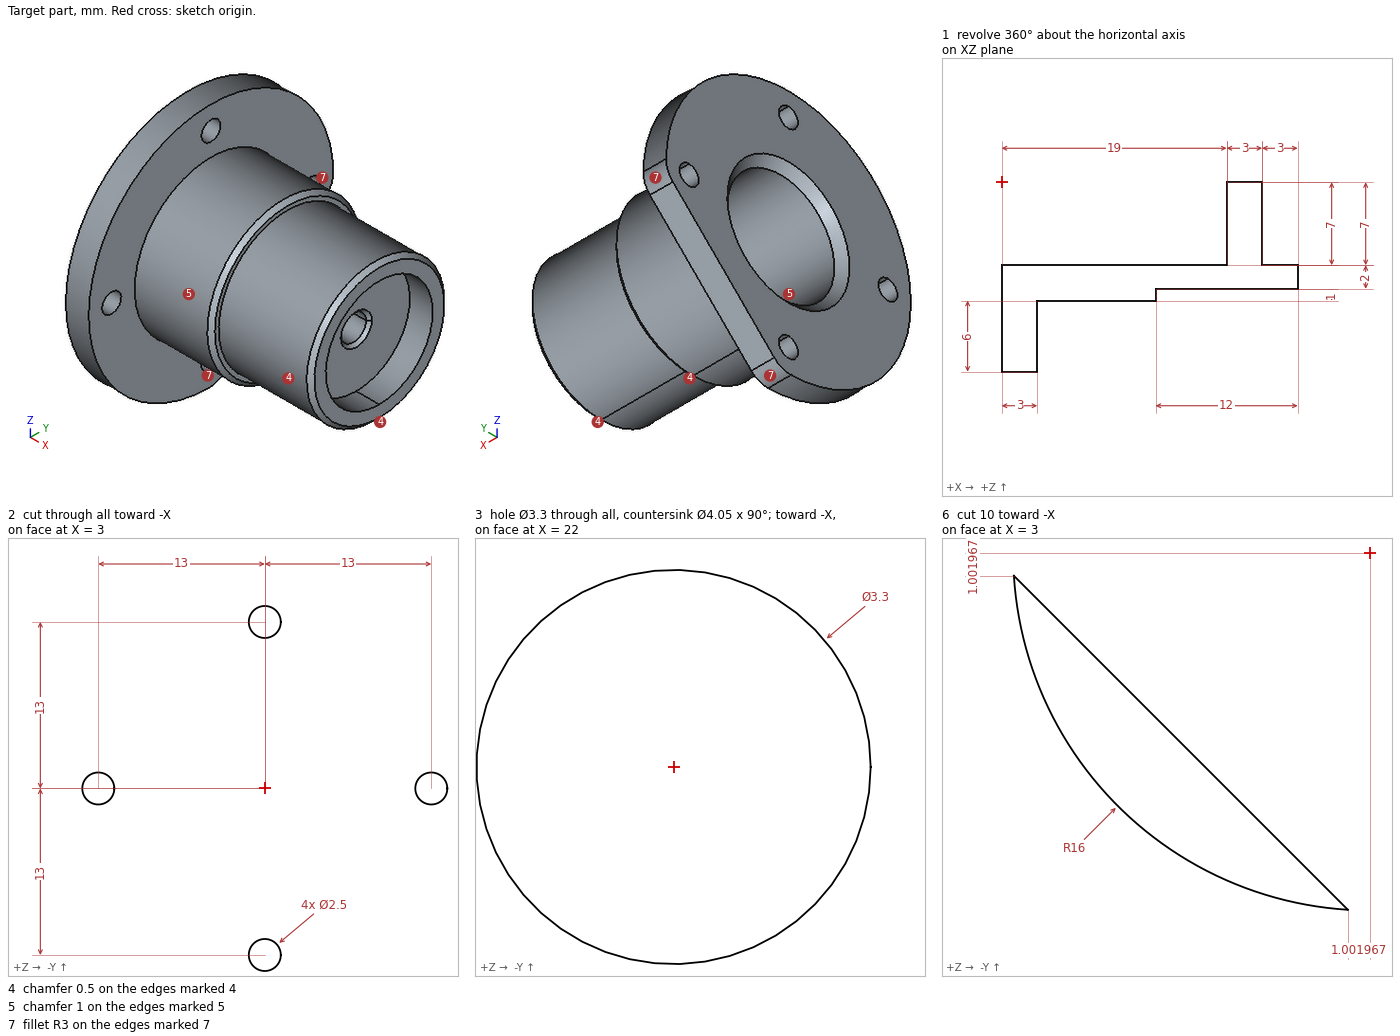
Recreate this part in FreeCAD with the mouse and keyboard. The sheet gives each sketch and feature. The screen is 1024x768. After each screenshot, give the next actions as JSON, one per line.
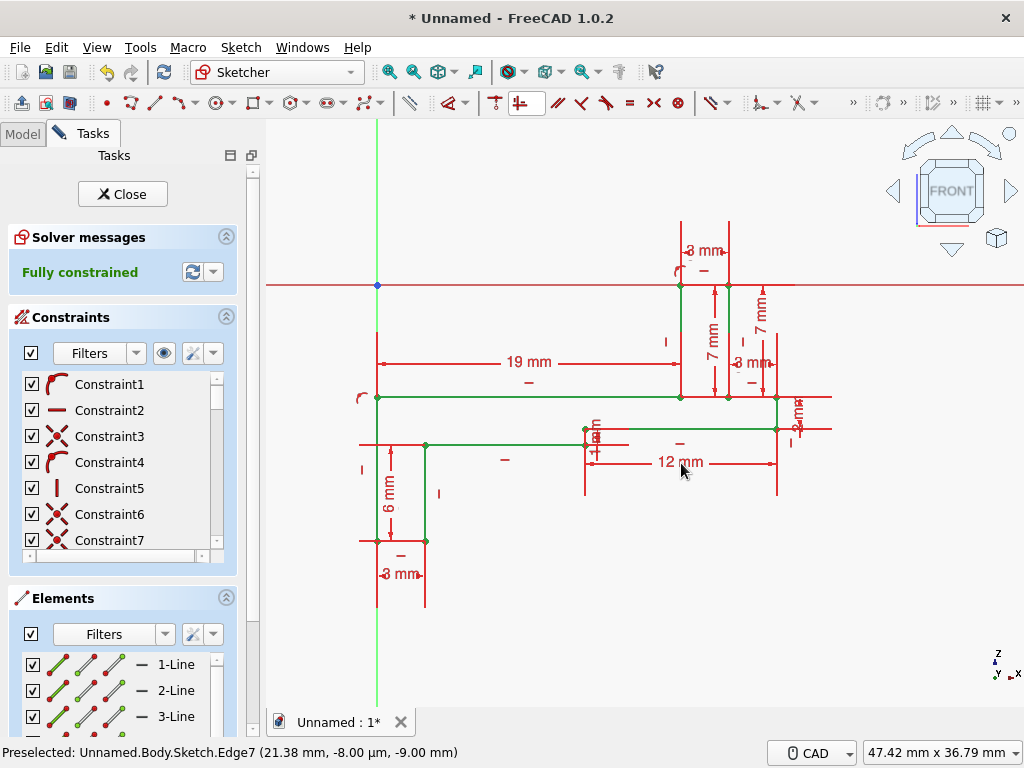
{"action": "left_click", "coordinate": [123, 194]}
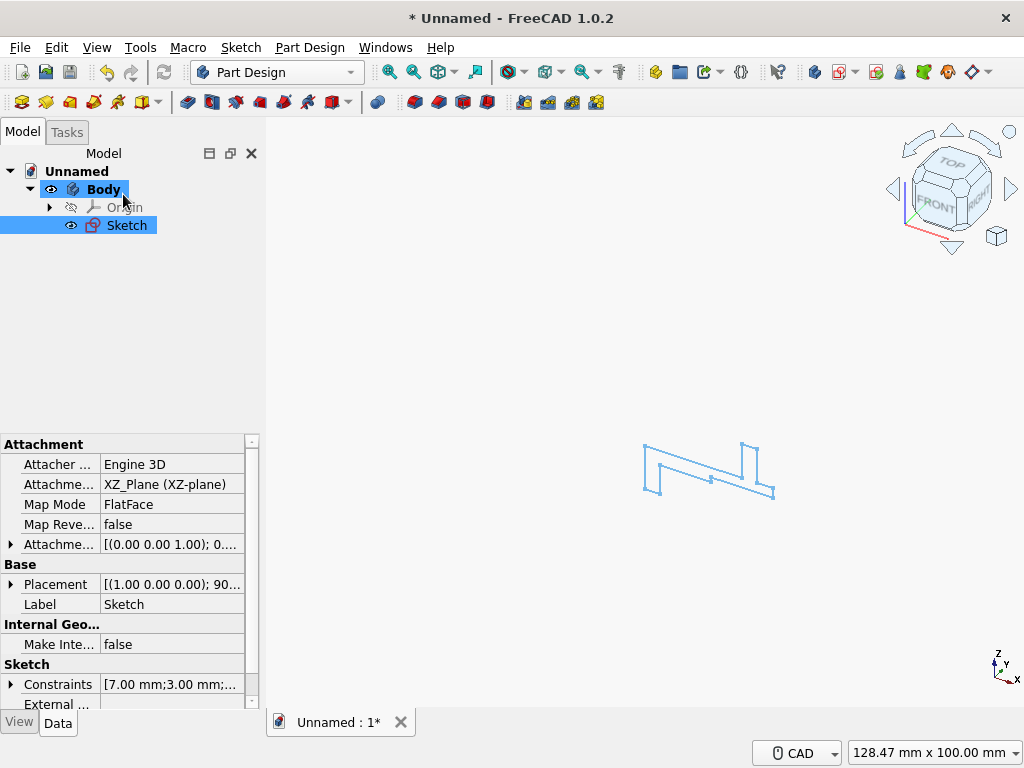
{"action": "left_click", "coordinate": [46, 102]}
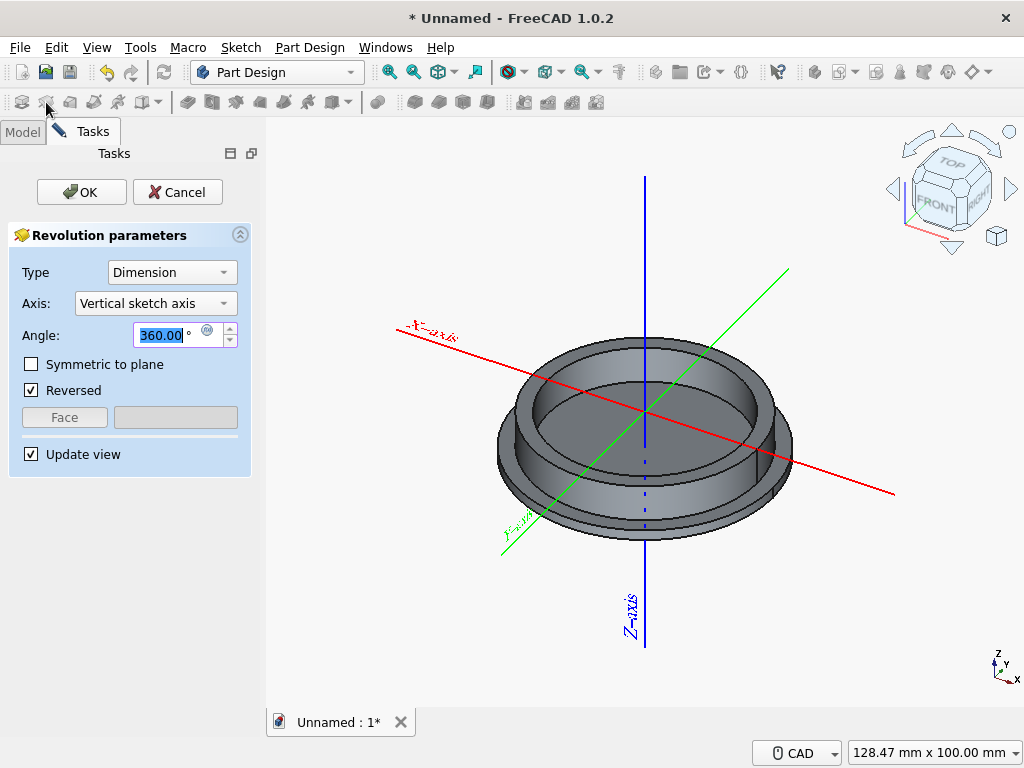
{"action": "left_click", "coordinate": [156, 304]}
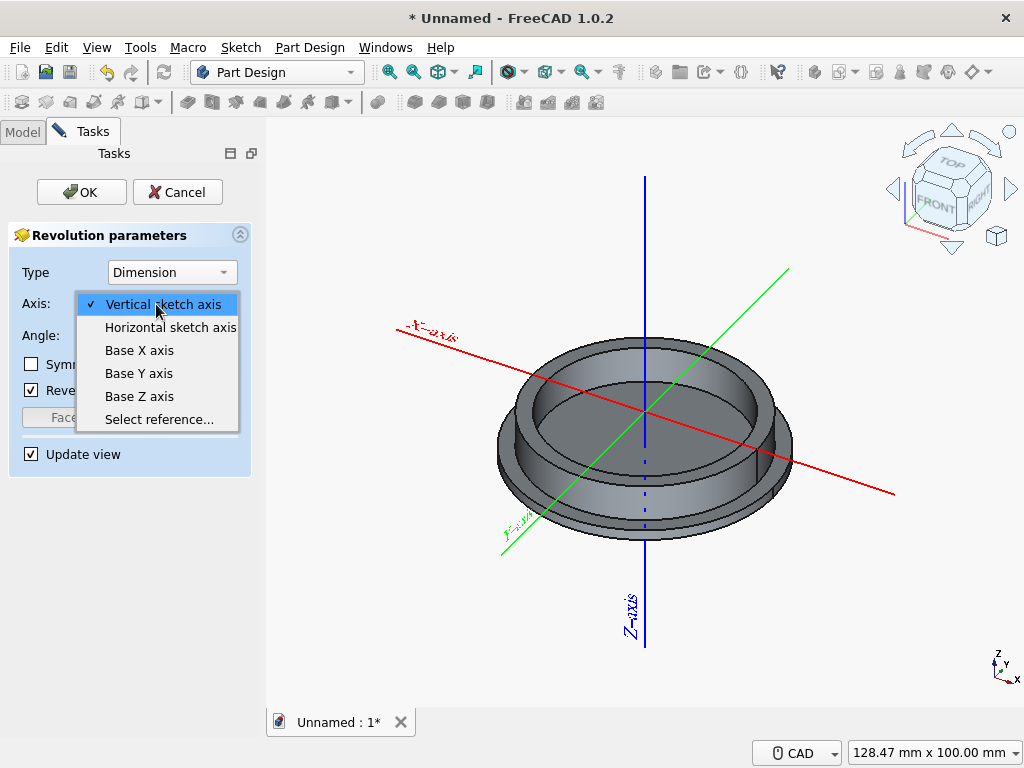
{"action": "left_click", "coordinate": [156, 328]}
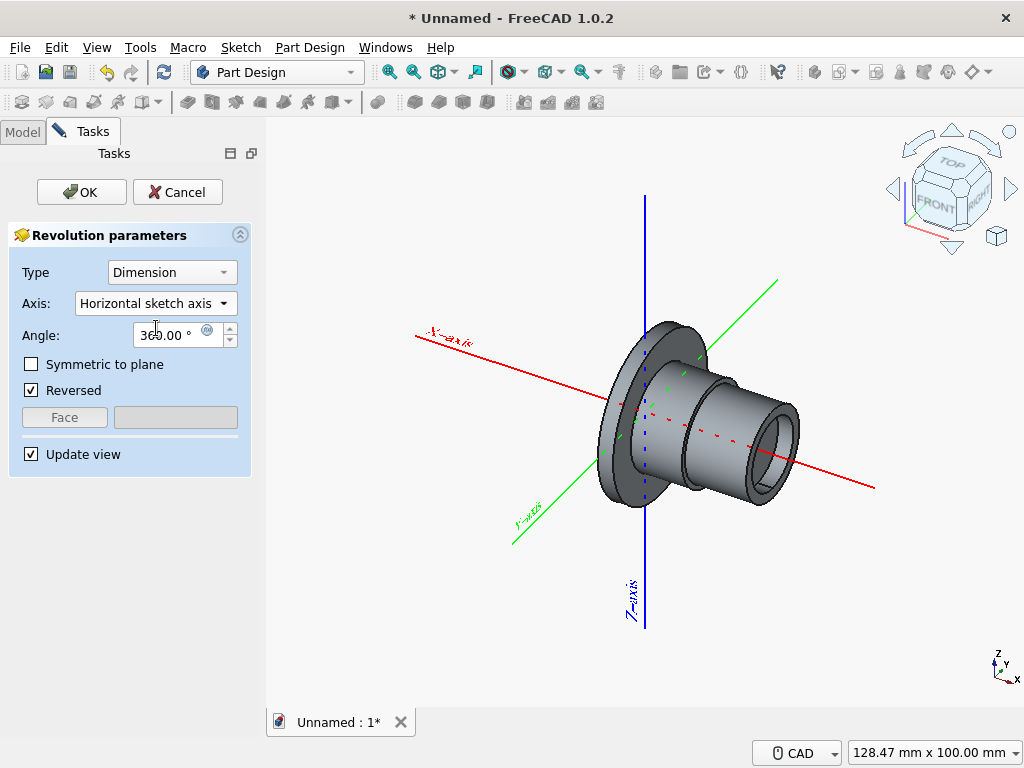
{"action": "left_click", "coordinate": [82, 192]}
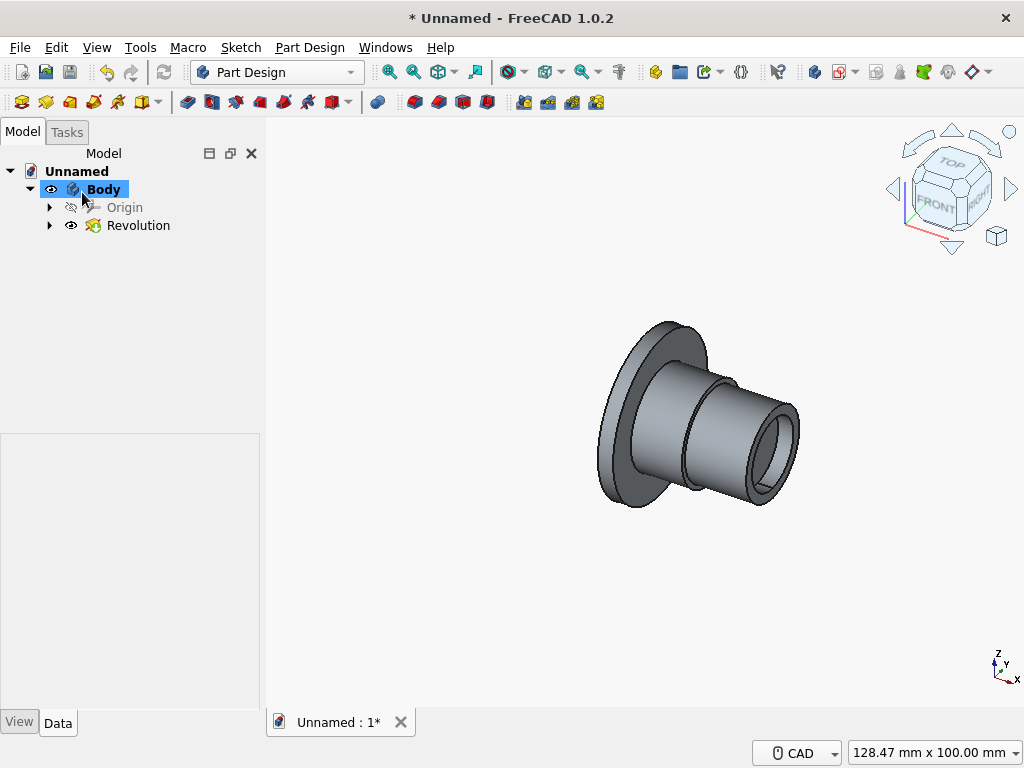
{"action": "left_click", "coordinate": [633, 487]}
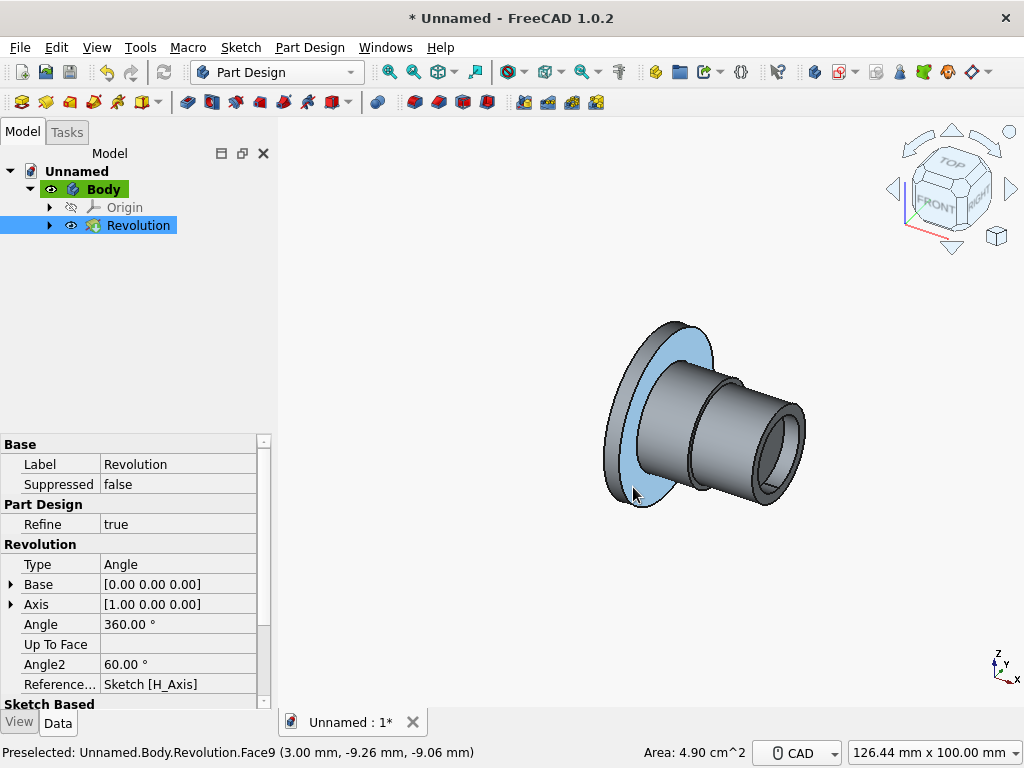
{"action": "left_click", "coordinate": [840, 72]}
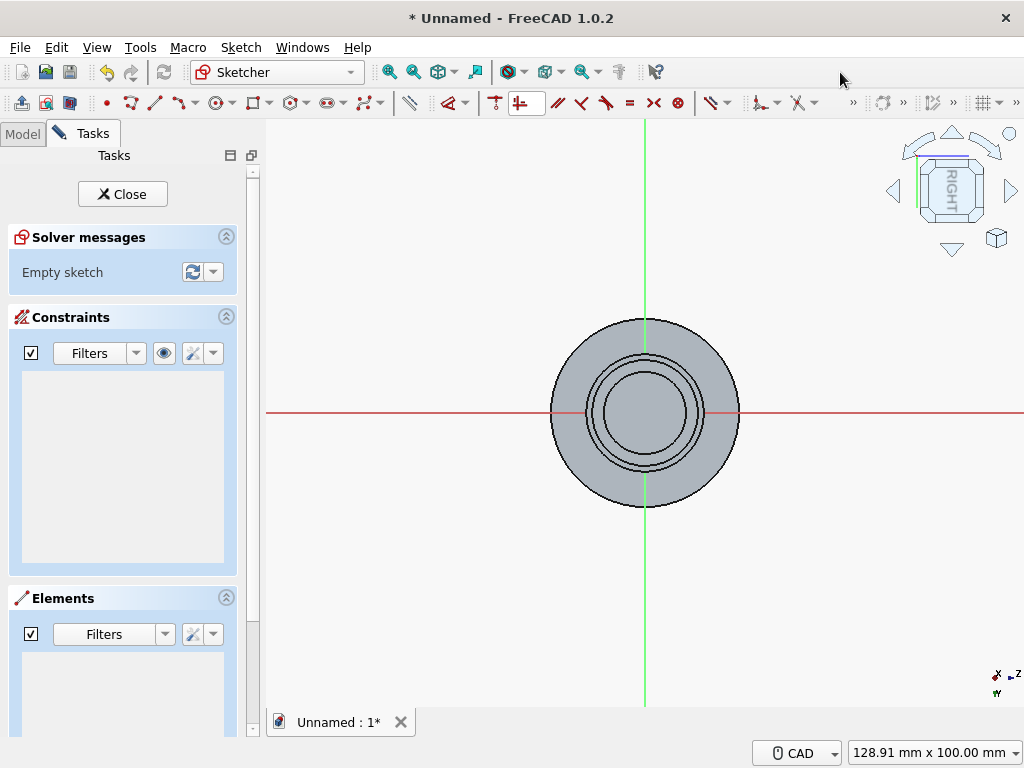
{"action": "scroll", "coordinate": [701, 413], "scroll_direction": "up", "scroll_amount": 4}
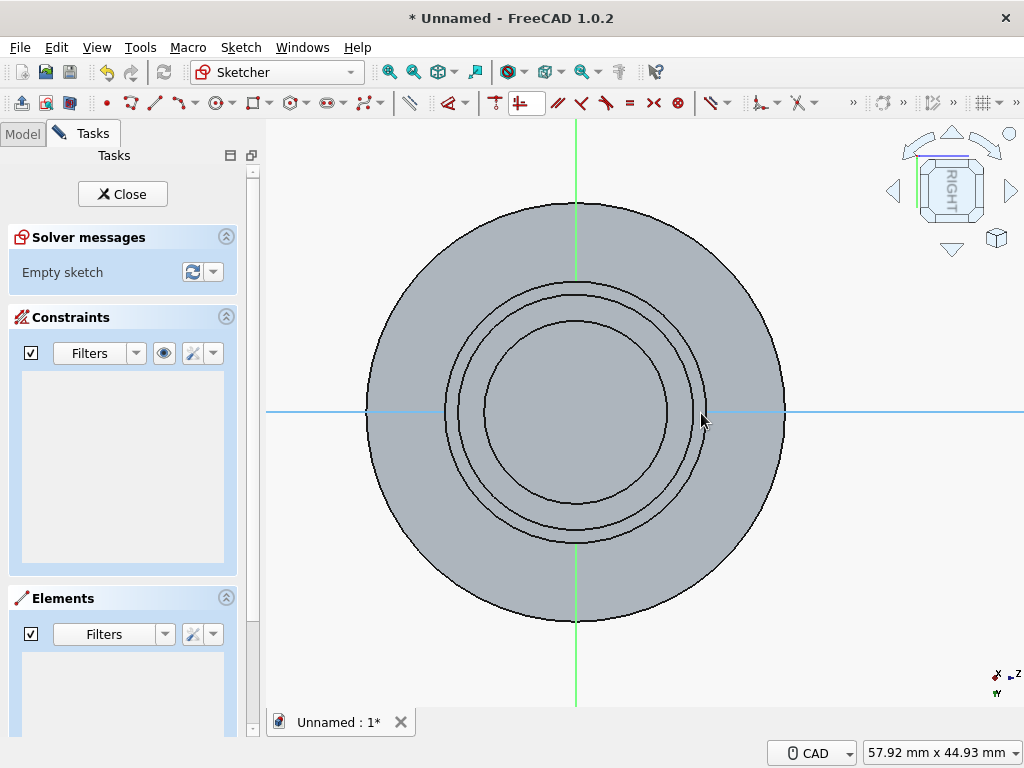
{"action": "left_click", "coordinate": [216, 104]}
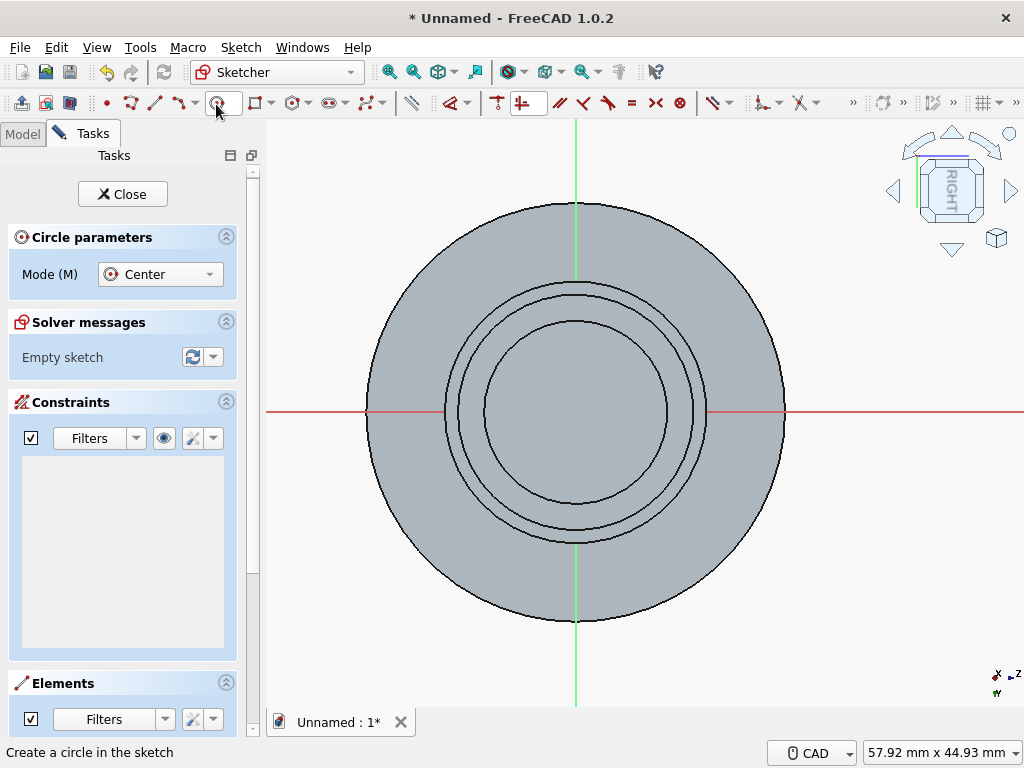
{"action": "scroll", "coordinate": [576, 583], "scroll_direction": "up", "scroll_amount": 2}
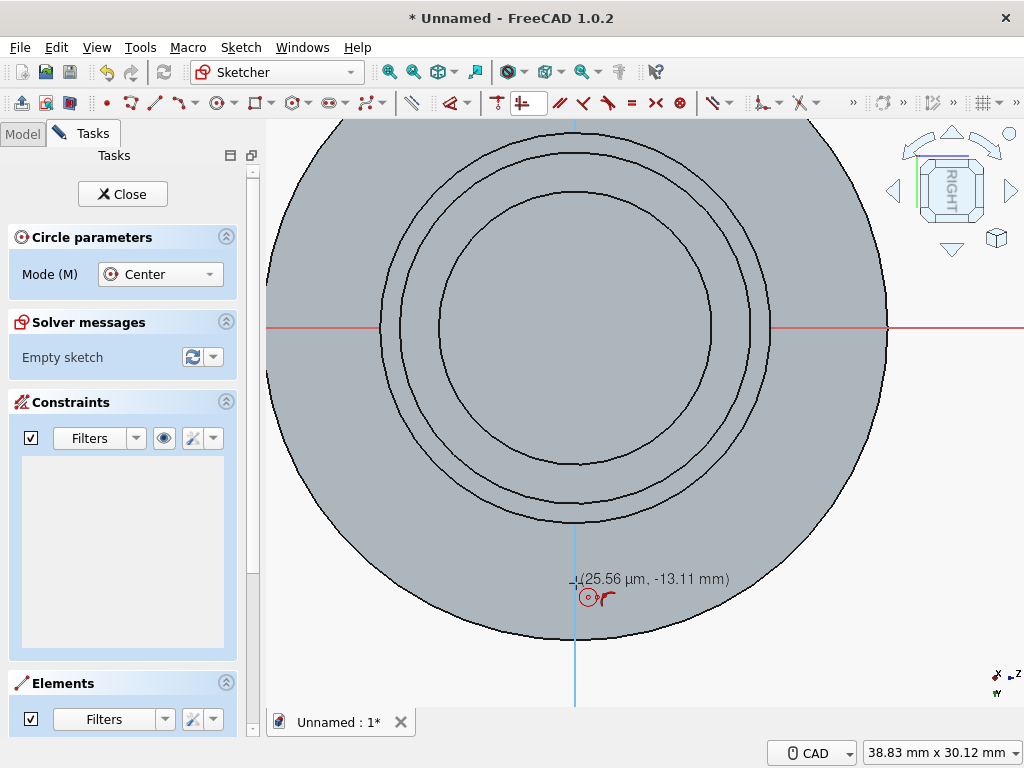
{"action": "left_click", "coordinate": [575, 582]}
{"action": "mouse_move", "coordinate": [593, 565]}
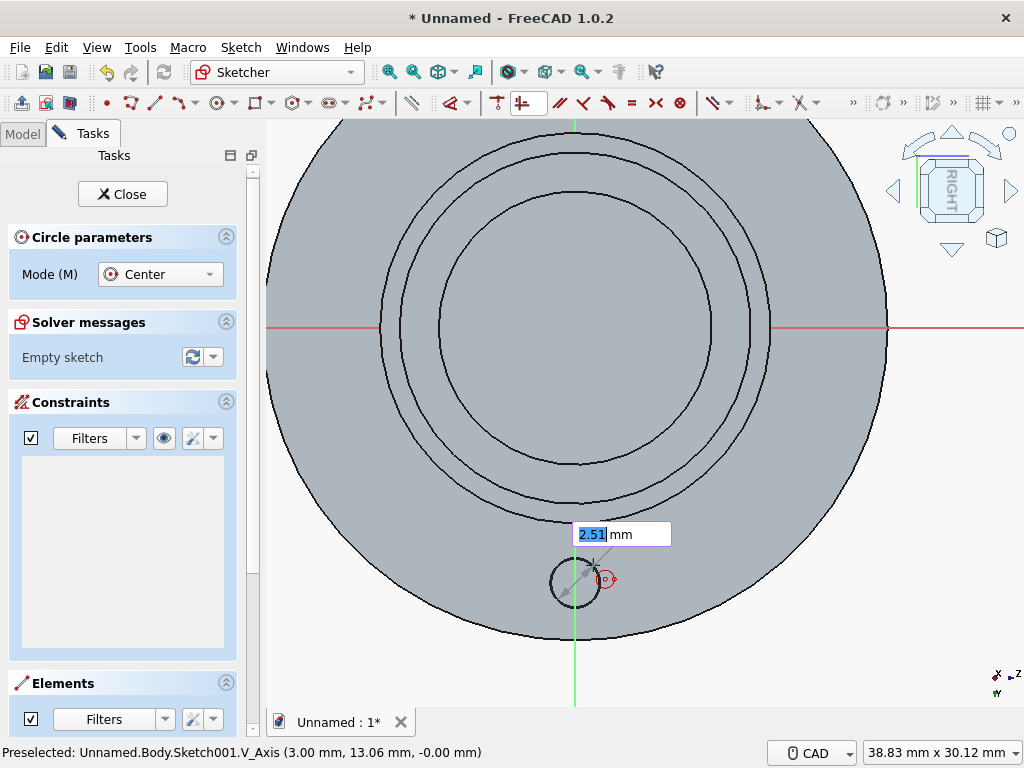
{"action": "type", "text": "2.5"}
{"action": "key", "text": "Return"}